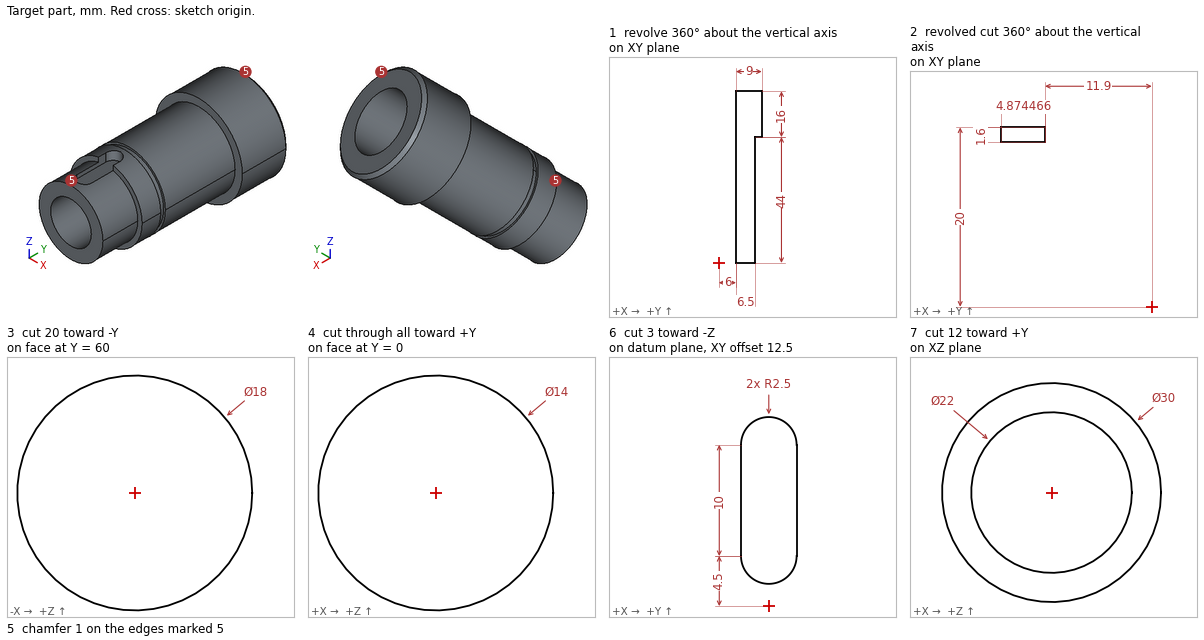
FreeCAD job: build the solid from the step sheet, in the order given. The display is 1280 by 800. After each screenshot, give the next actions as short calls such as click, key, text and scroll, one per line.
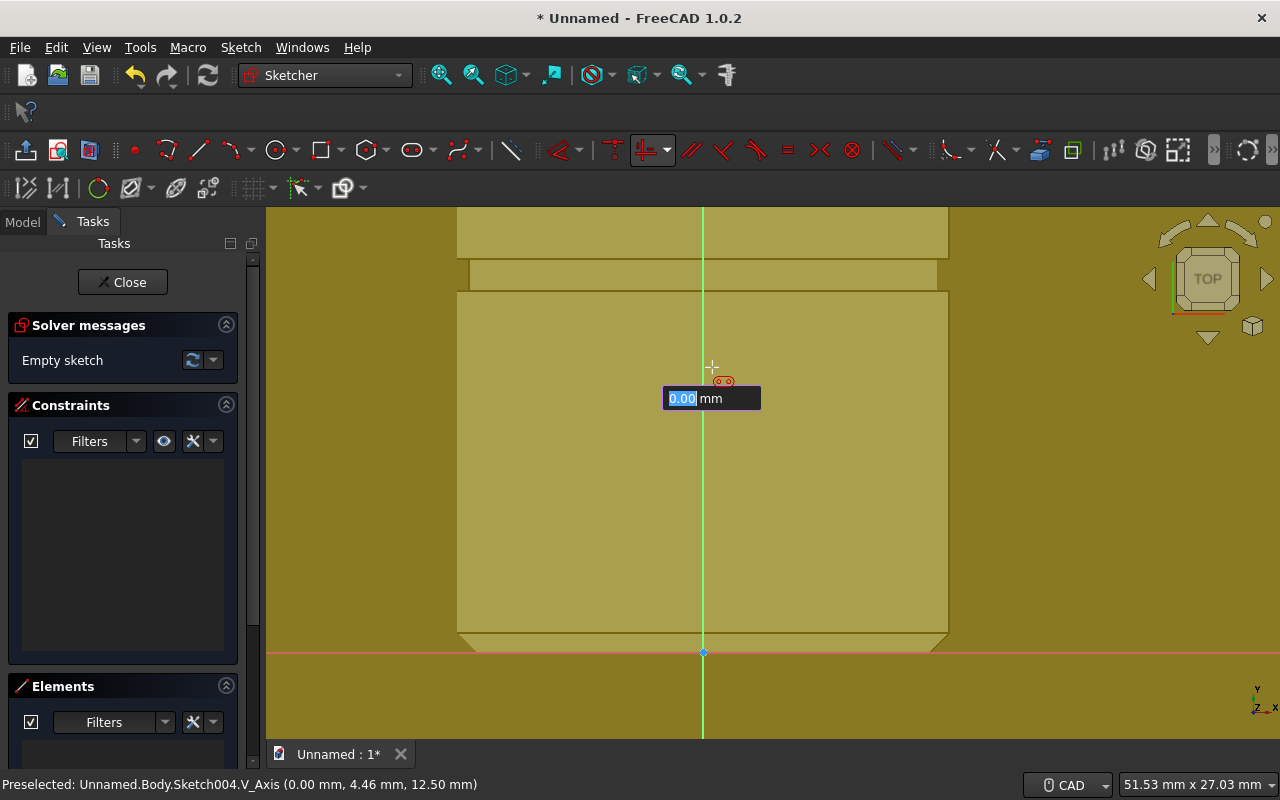
click(753, 466)
key(Escape)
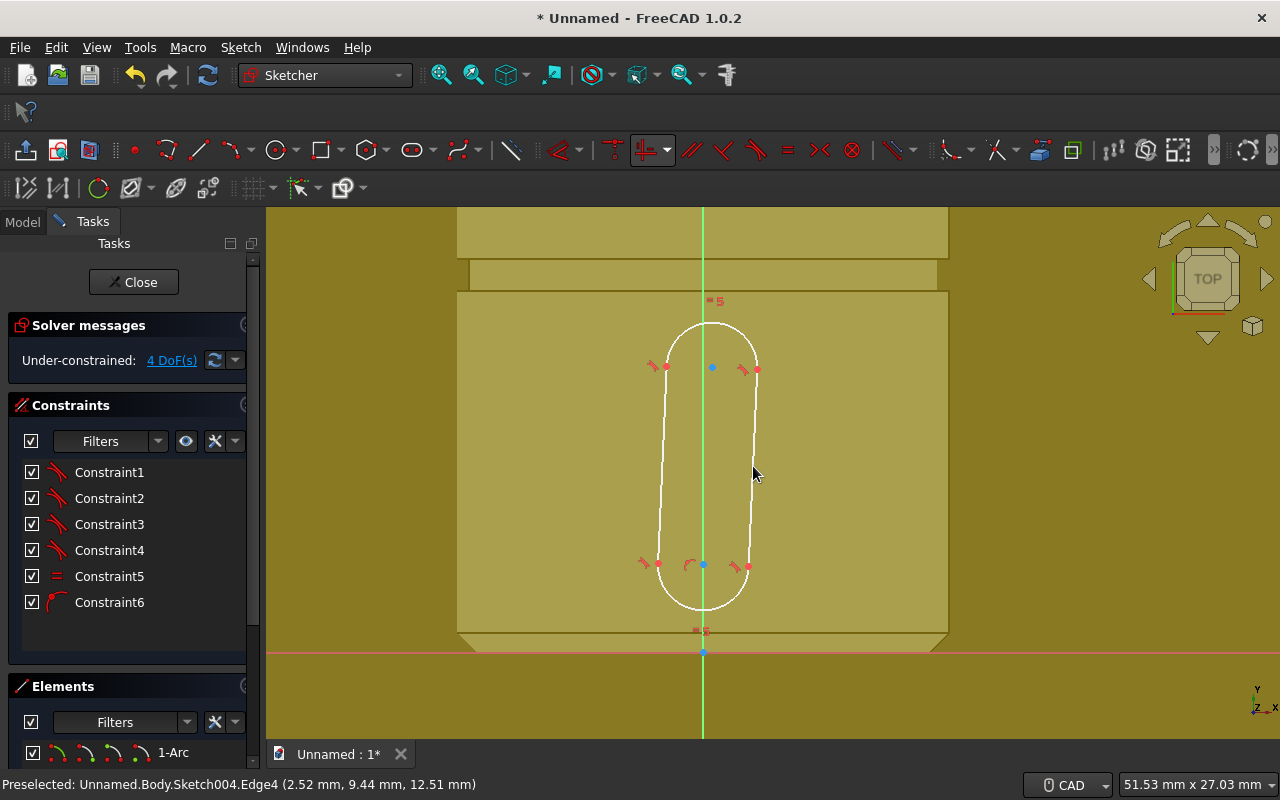
click(661, 504)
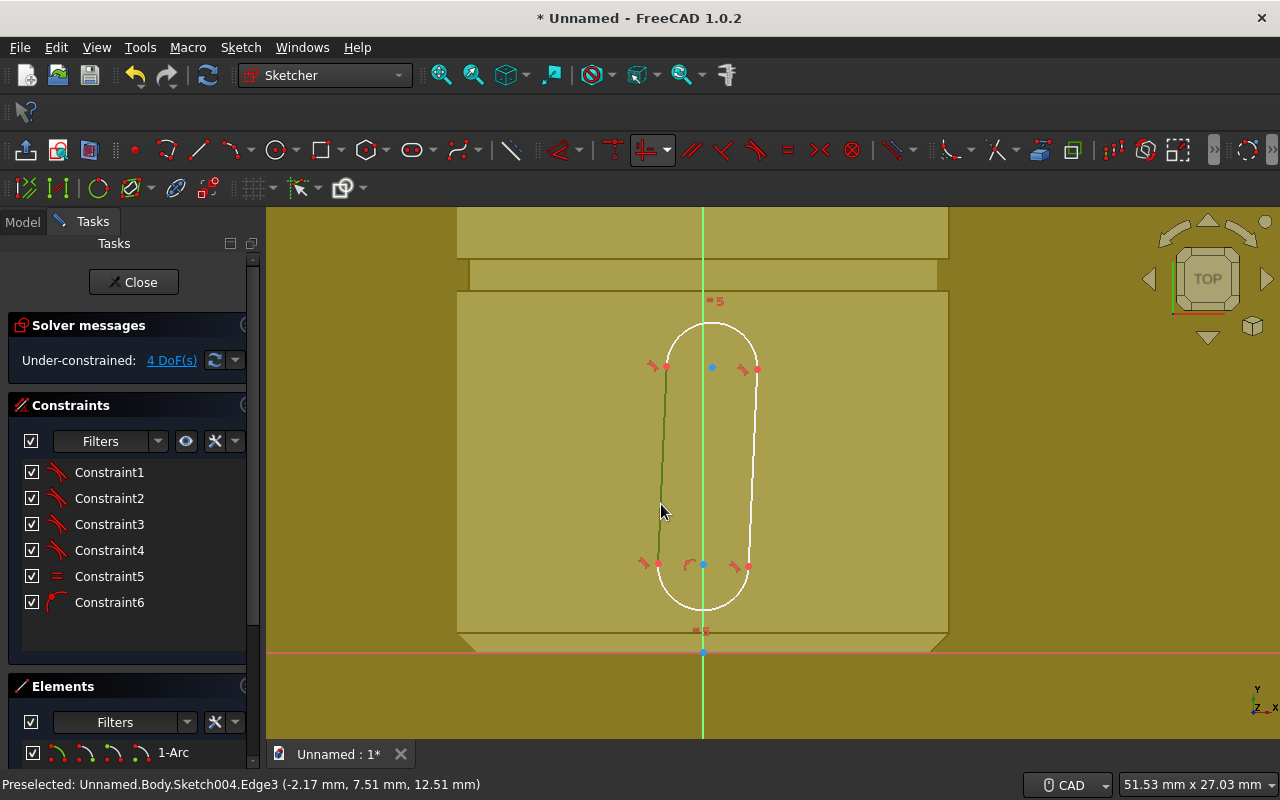
key(v)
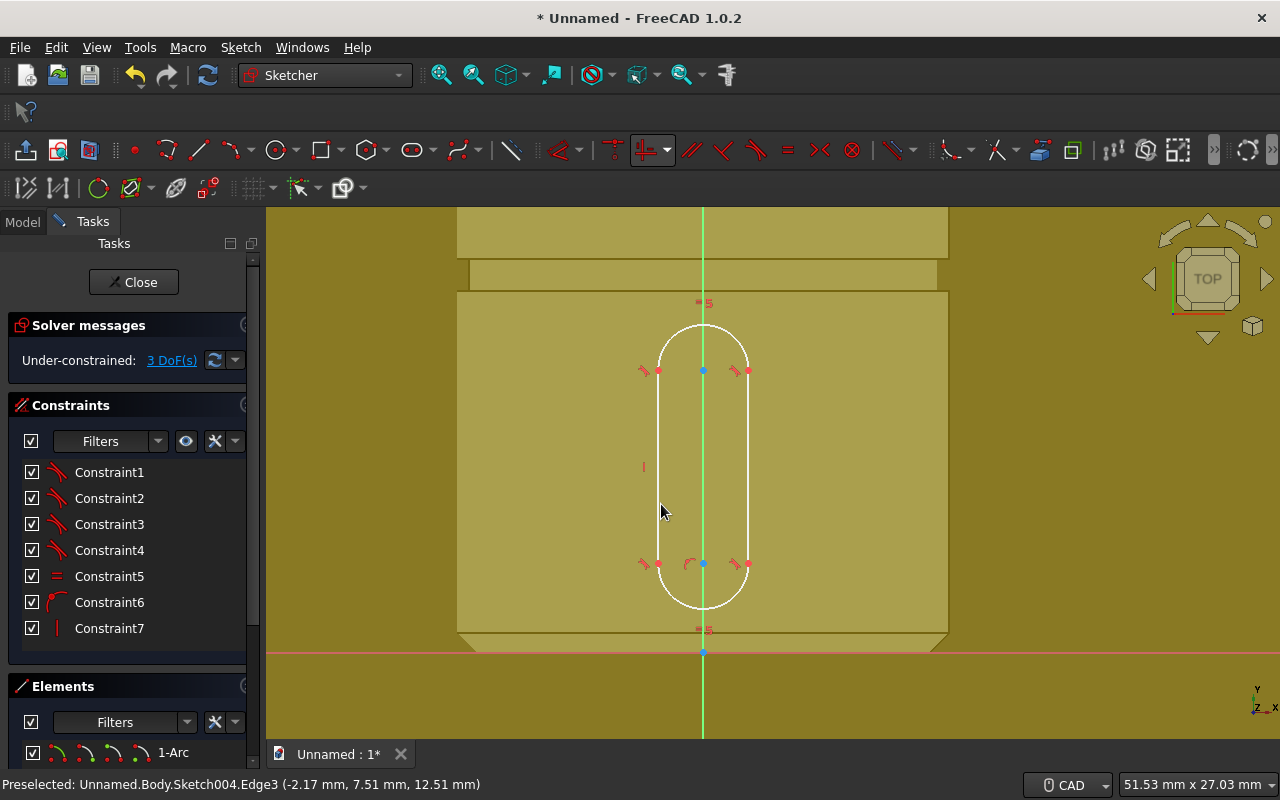
click(558, 150)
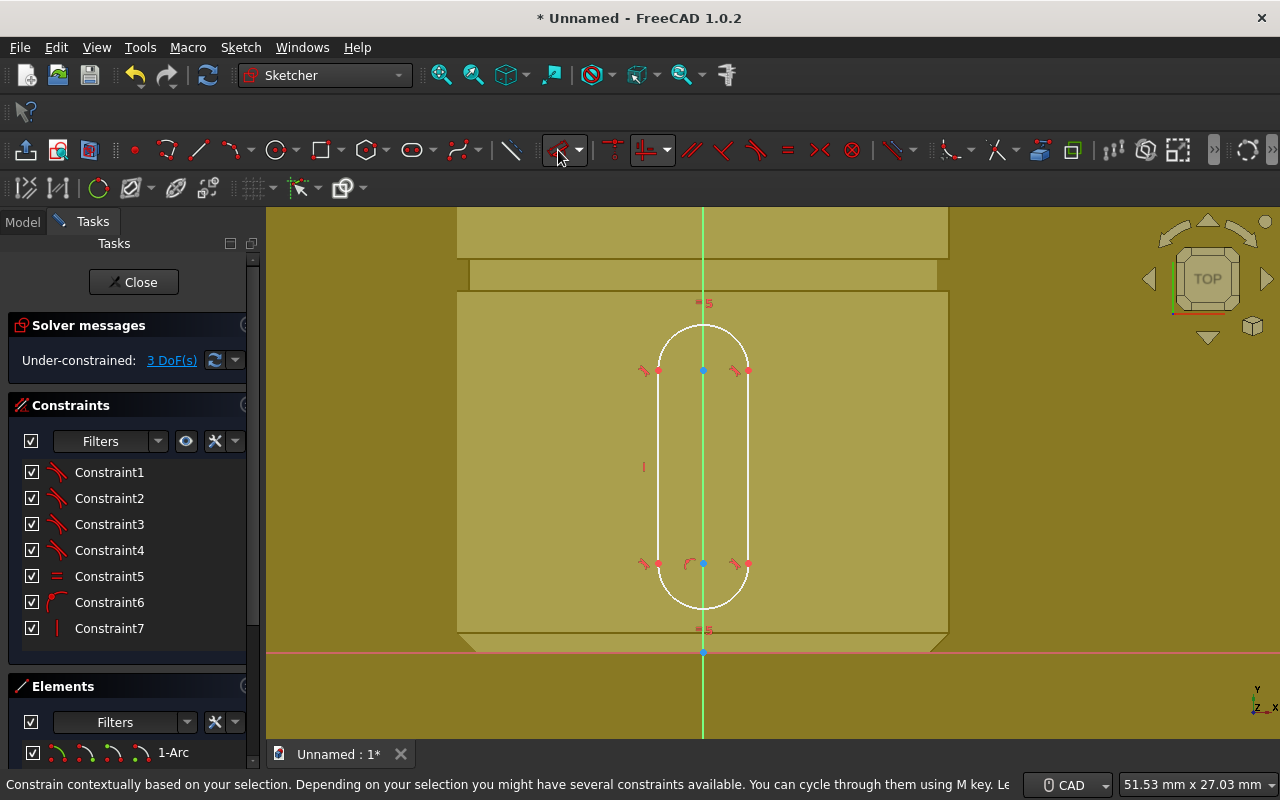
click(677, 600)
click(658, 626)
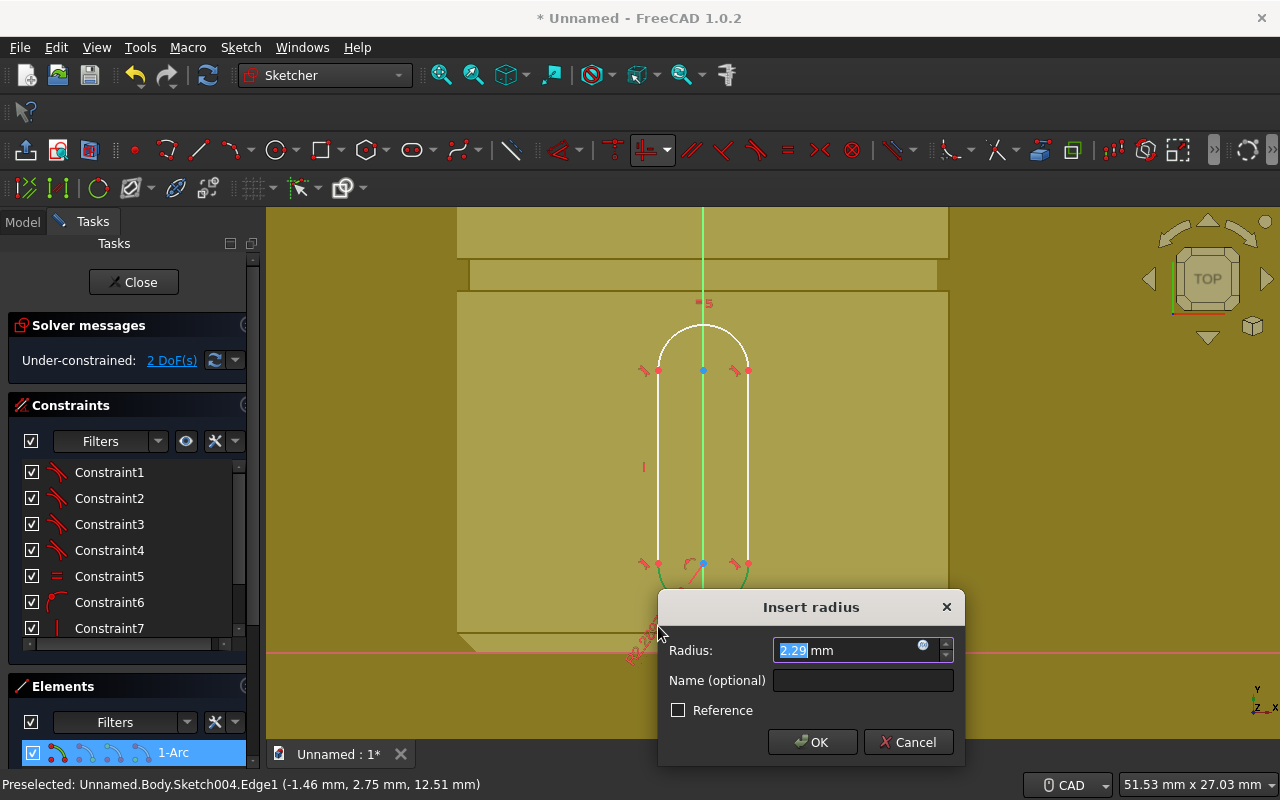
text(2.5)
key(Return)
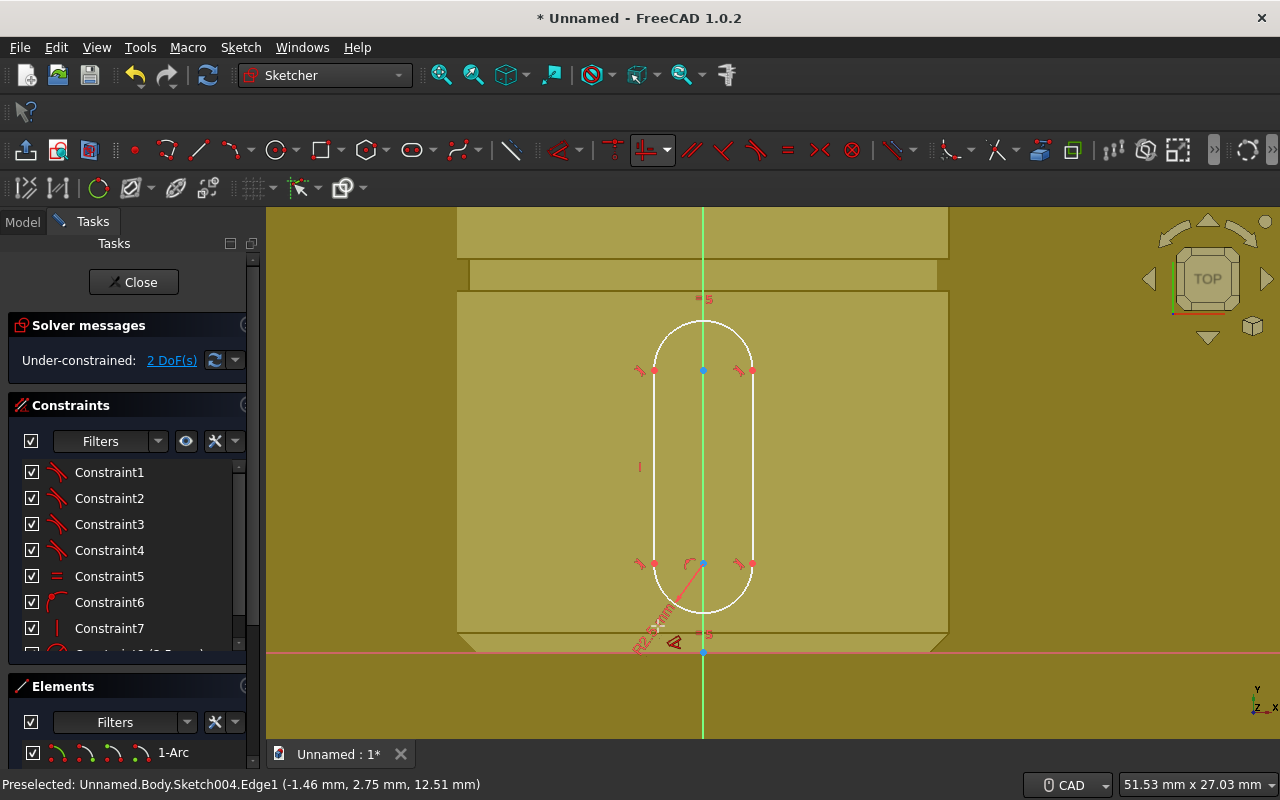
click(654, 506)
click(620, 467)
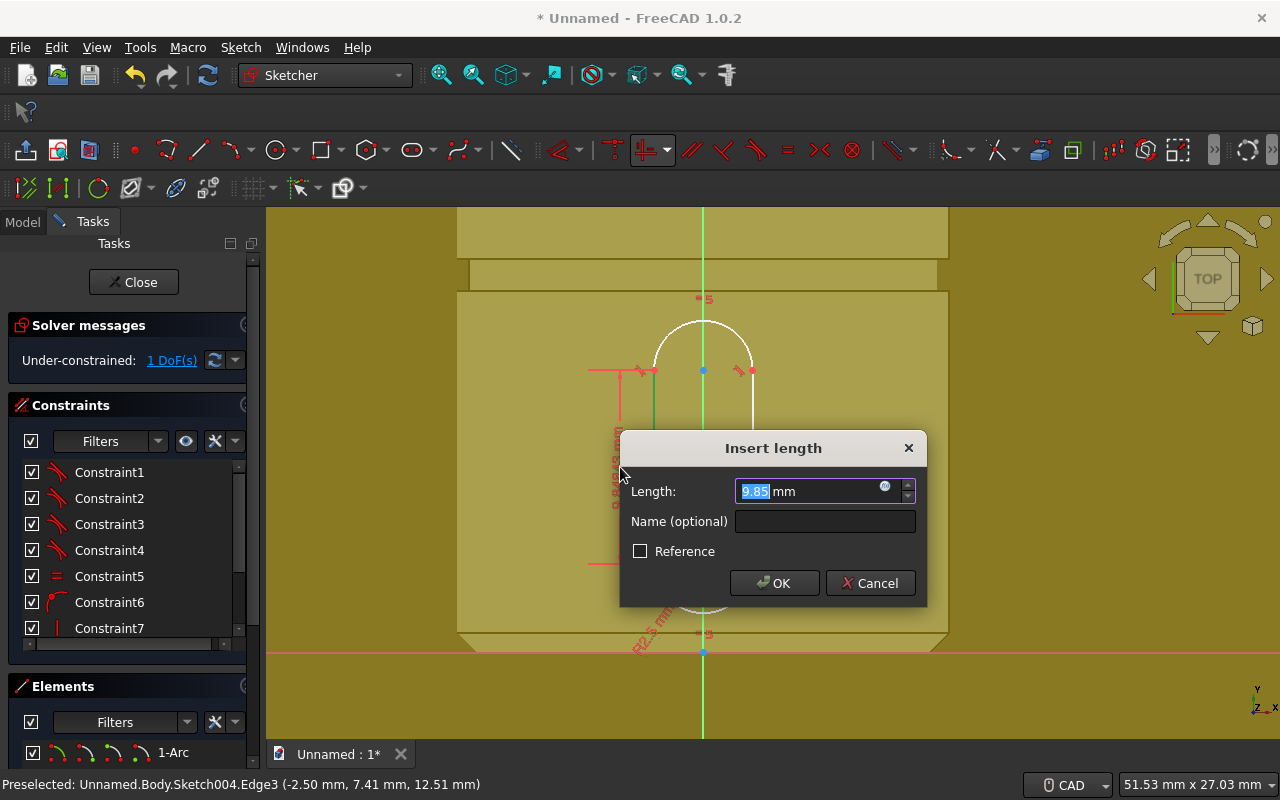
text(10)
key(Return)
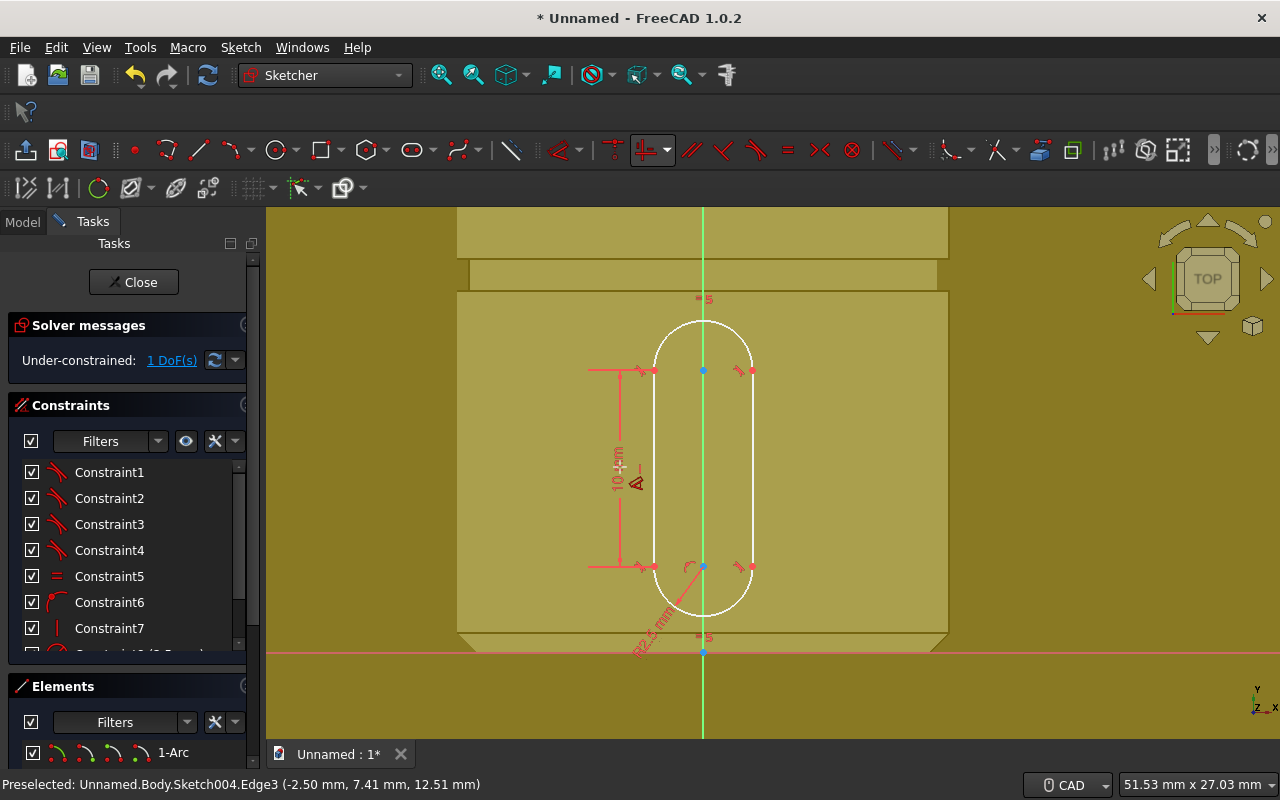
click(654, 567)
click(620, 590)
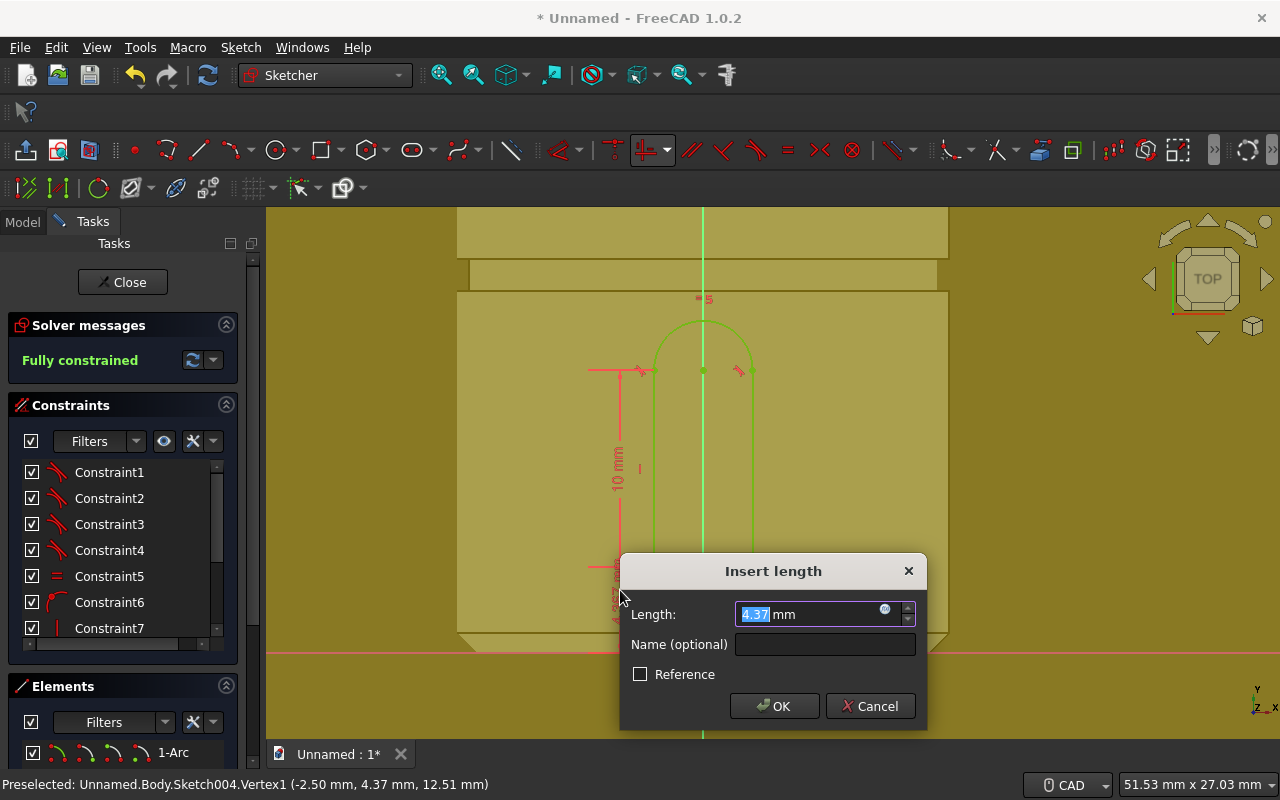
text(4.5)
key(Return)
key(Escape)